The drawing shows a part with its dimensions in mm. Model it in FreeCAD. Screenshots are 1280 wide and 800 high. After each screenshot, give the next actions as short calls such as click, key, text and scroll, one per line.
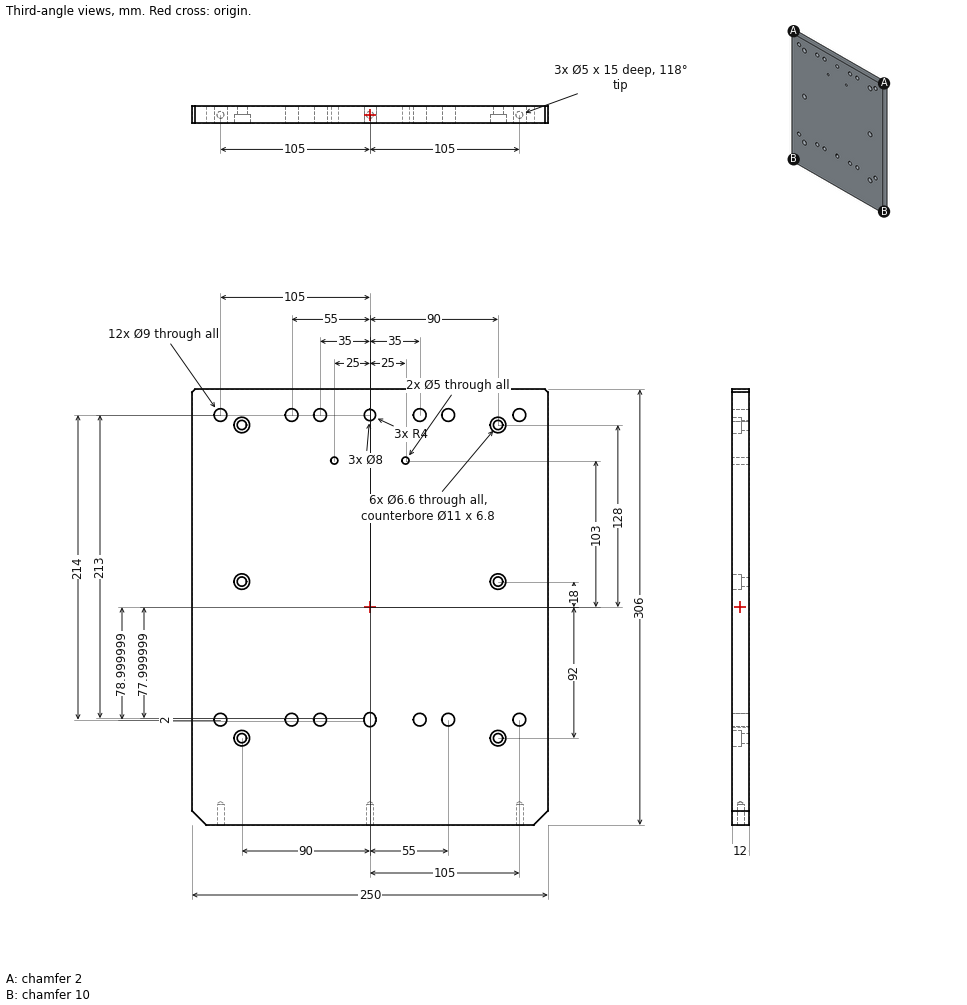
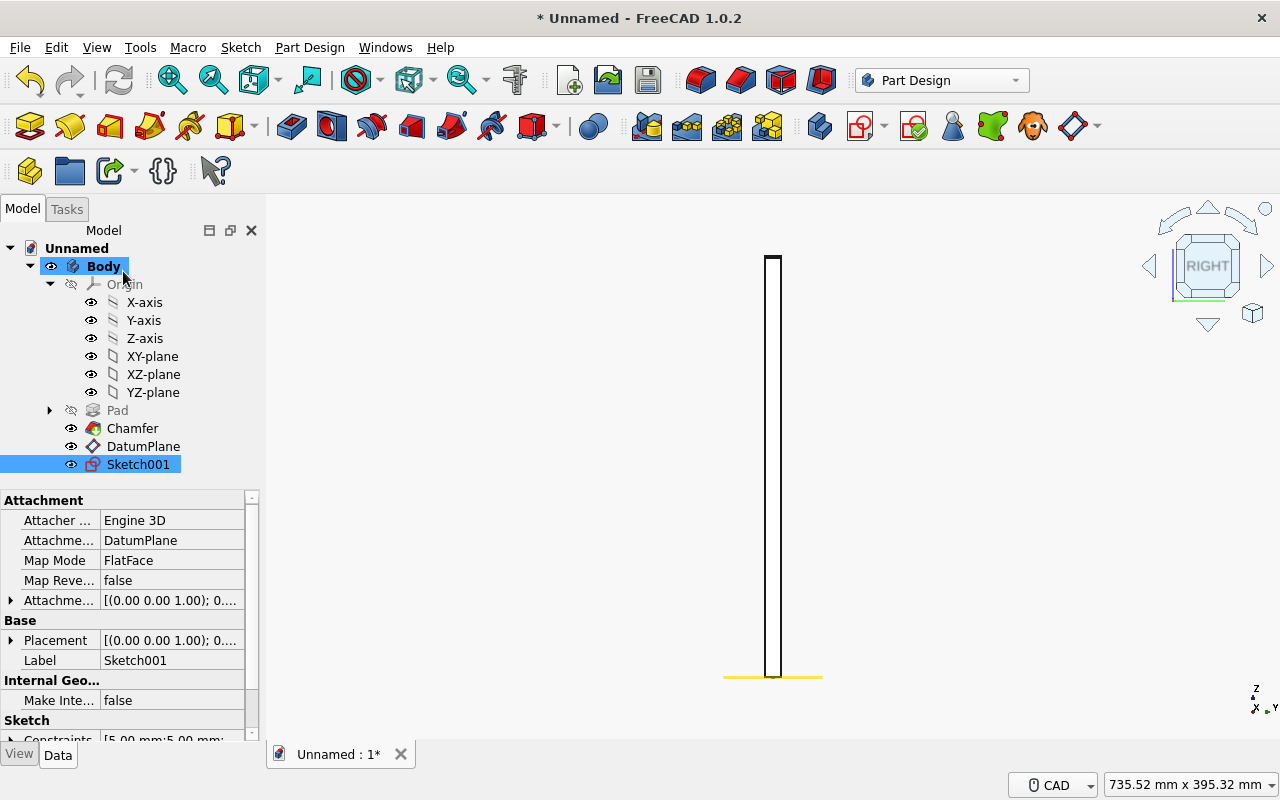
click(332, 126)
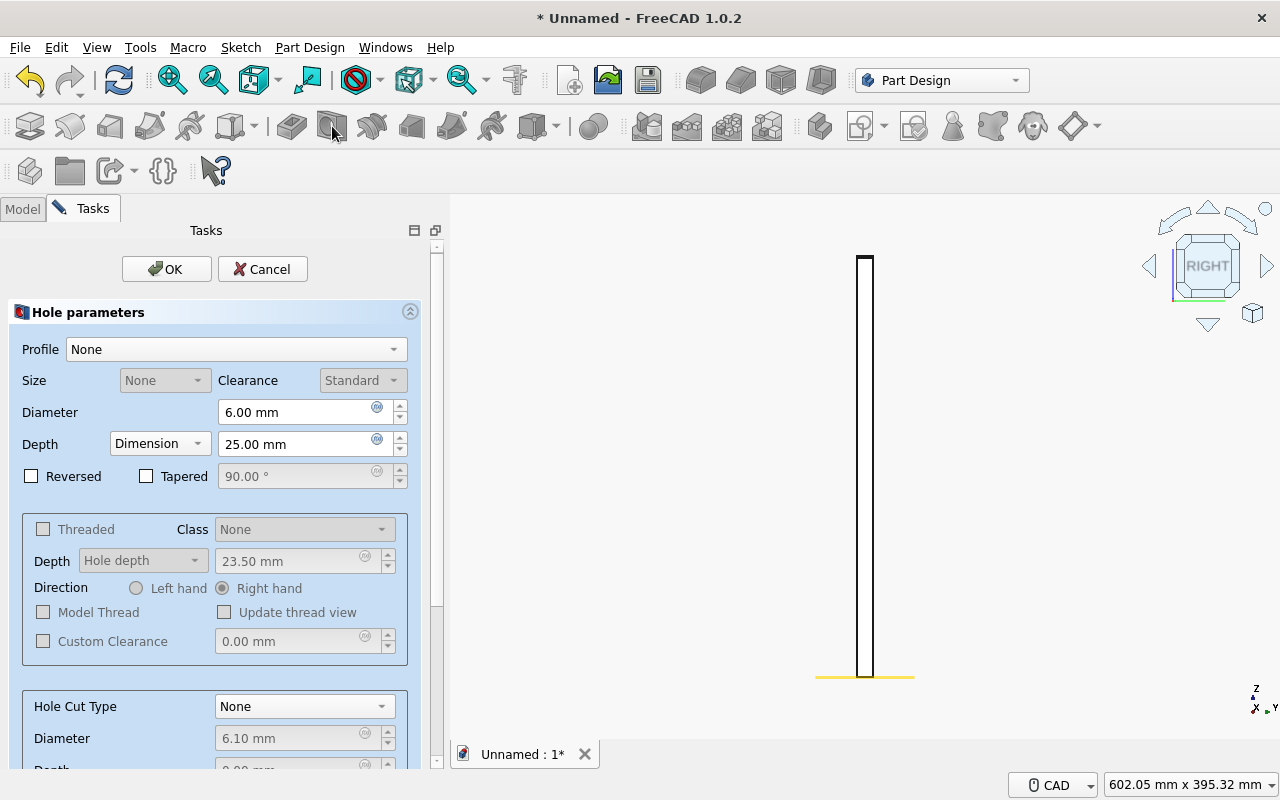
triple_click(305, 412)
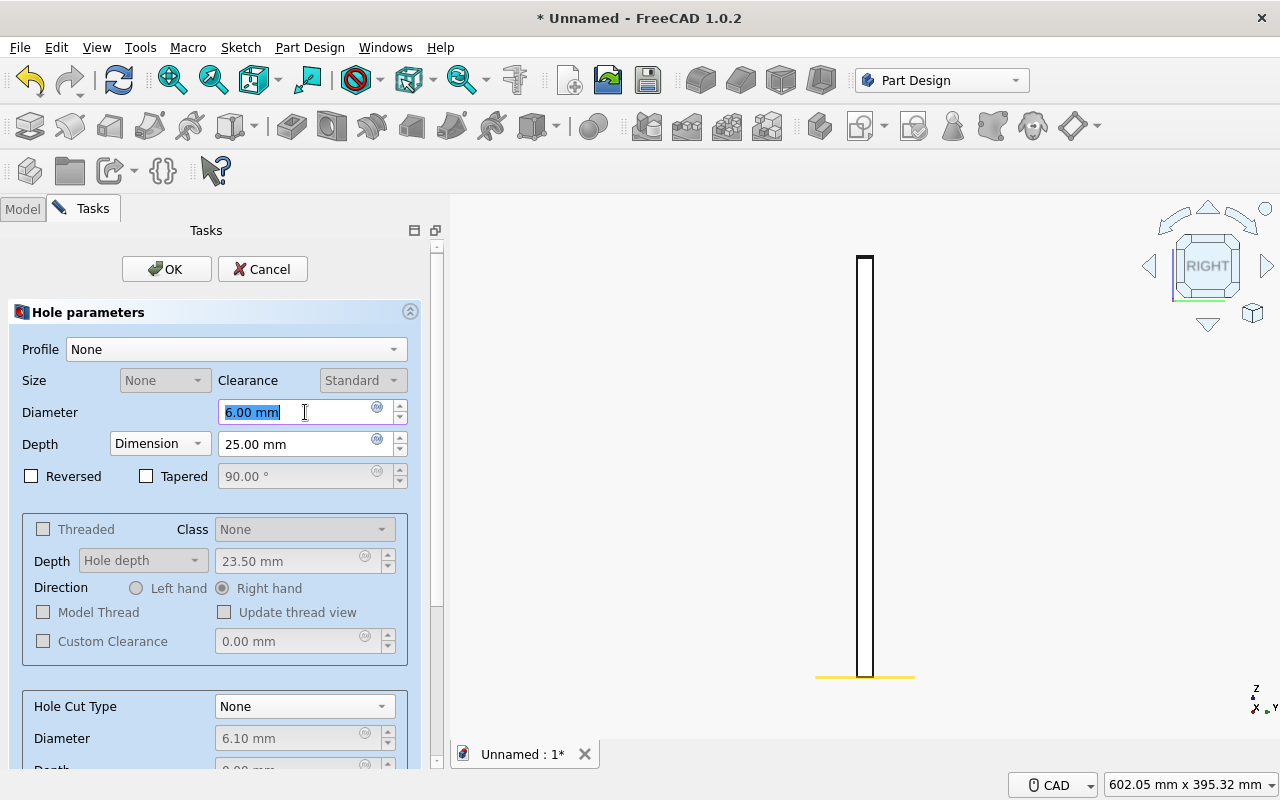
text(5)
key(Tab)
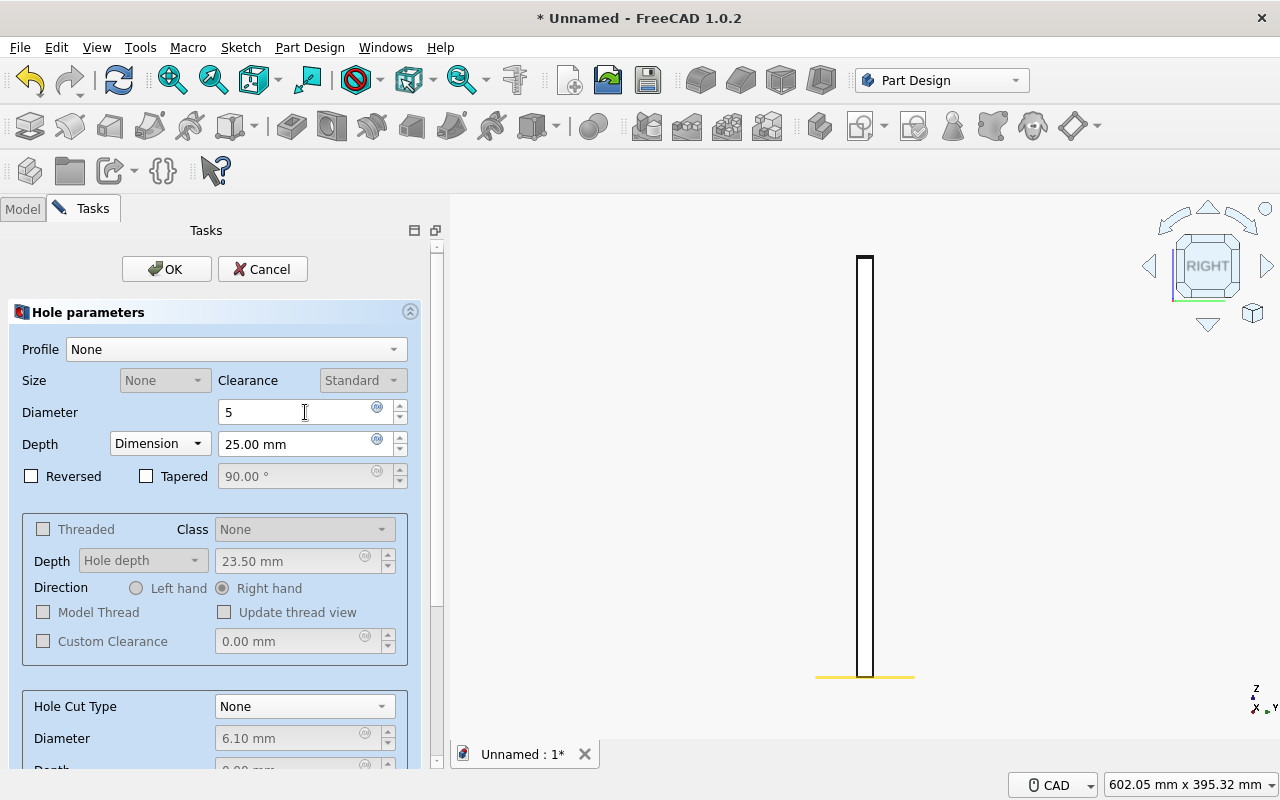
triple_click(305, 444)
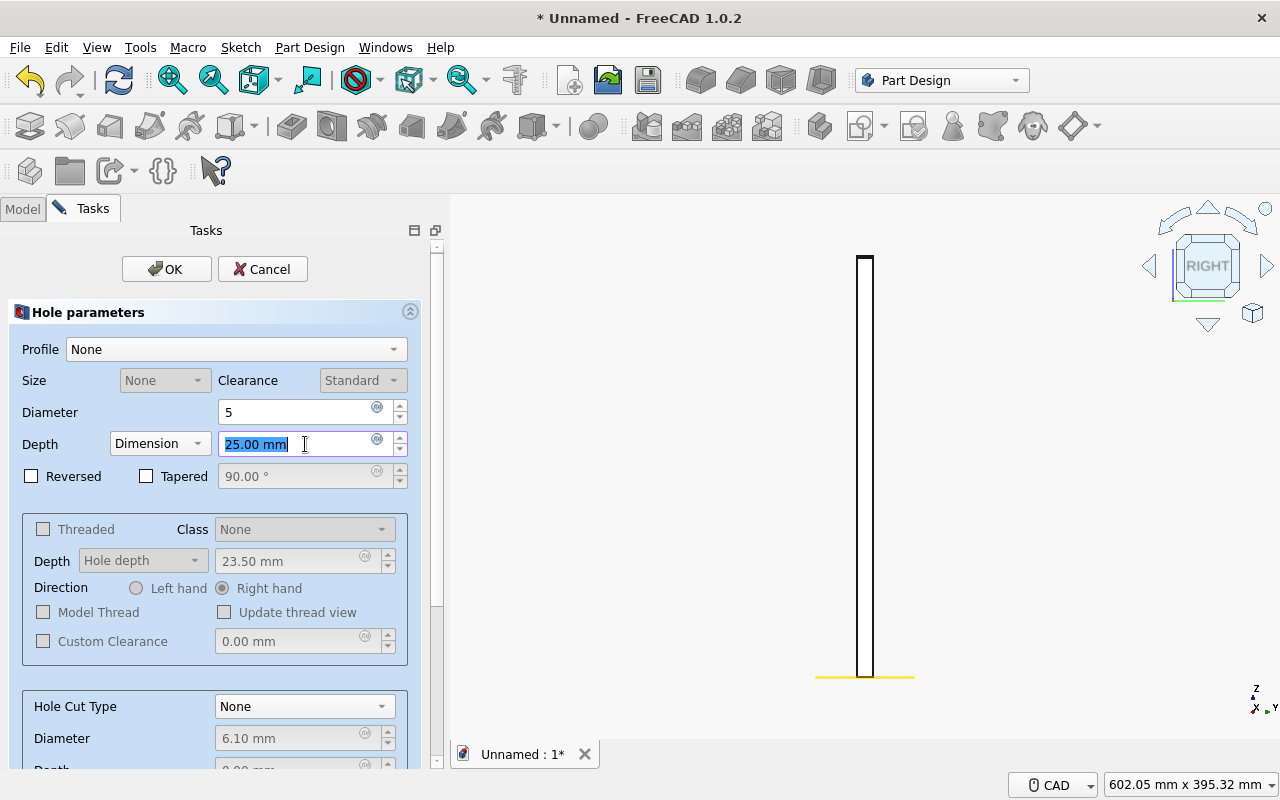
text(15)
key(Tab)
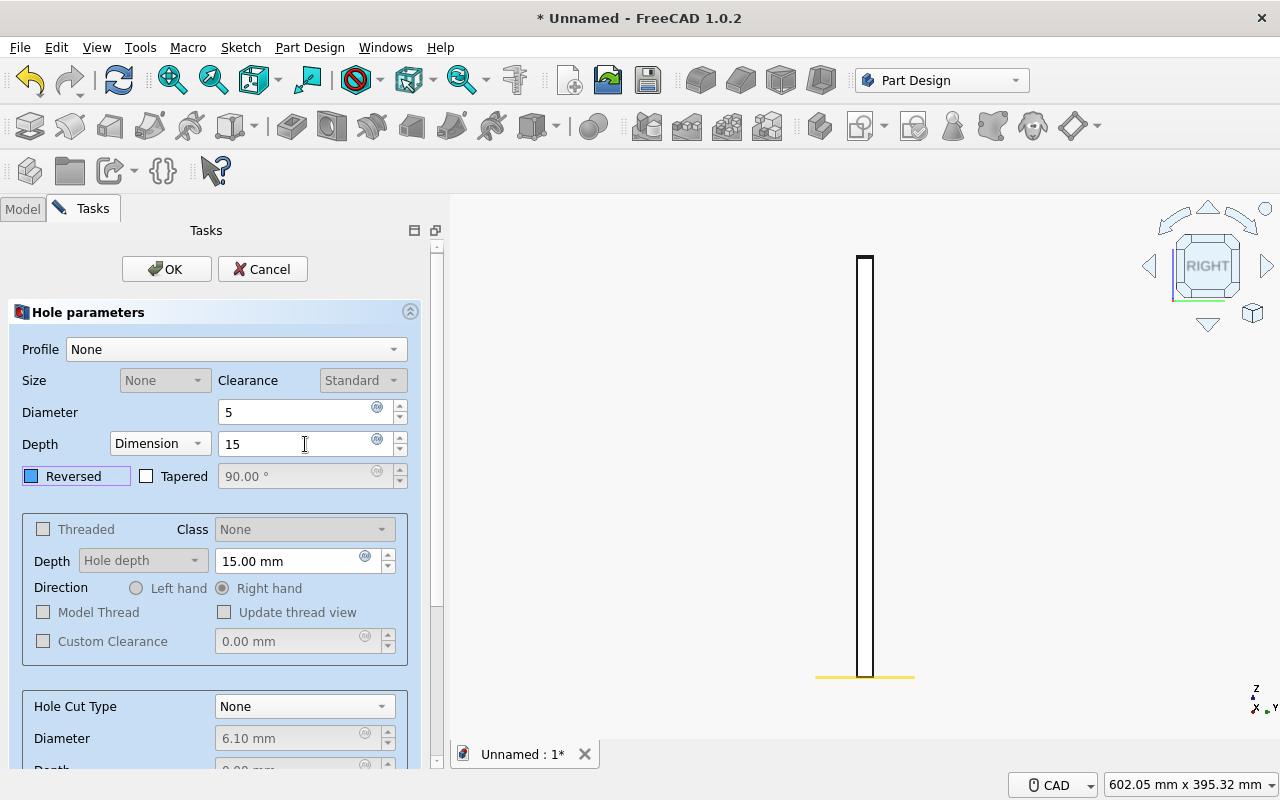
click(30, 476)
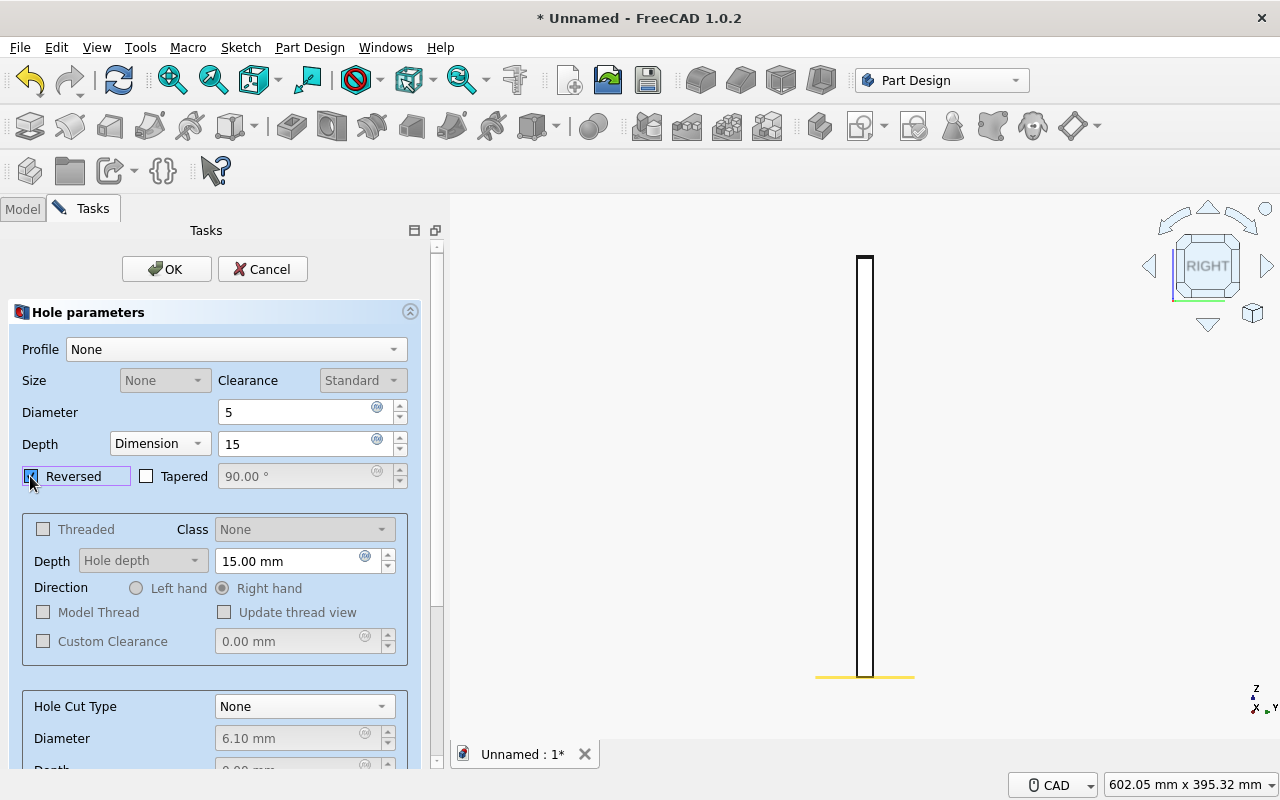
click(167, 269)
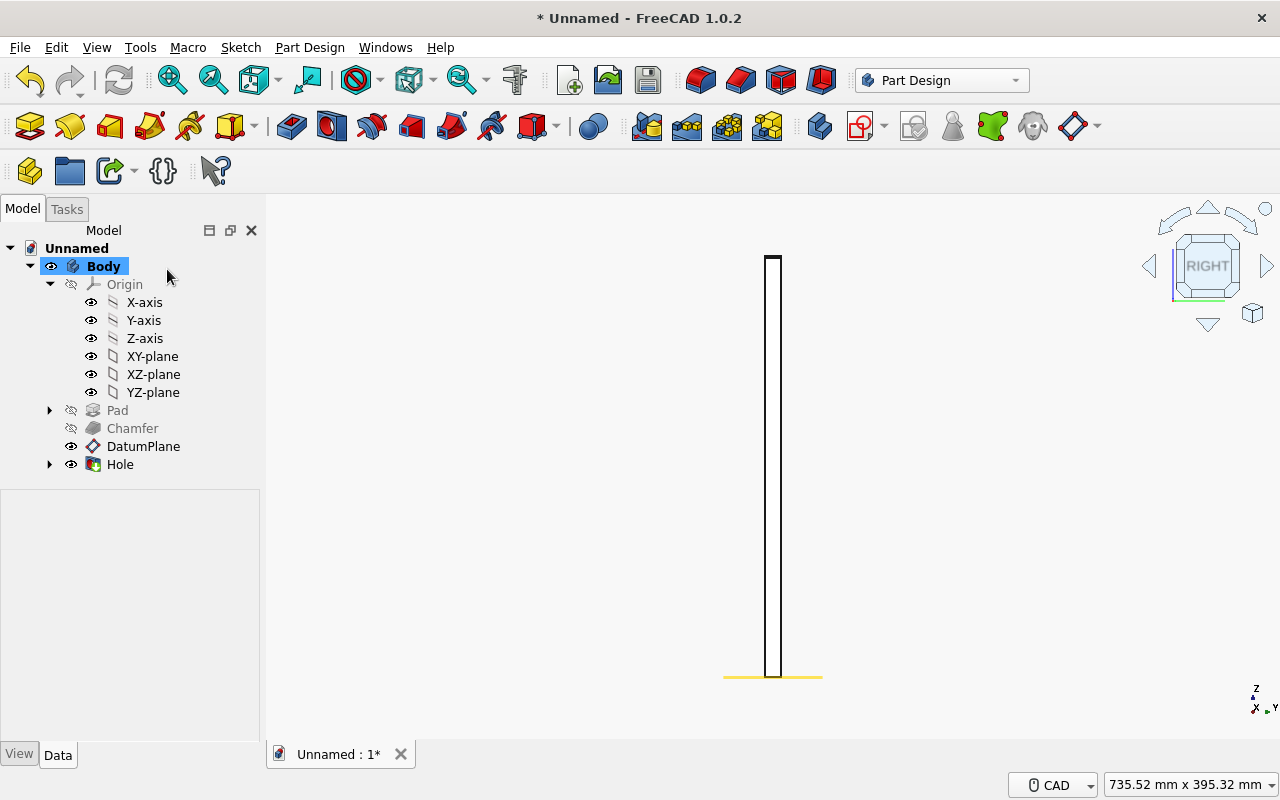
click(116, 446)
key(space)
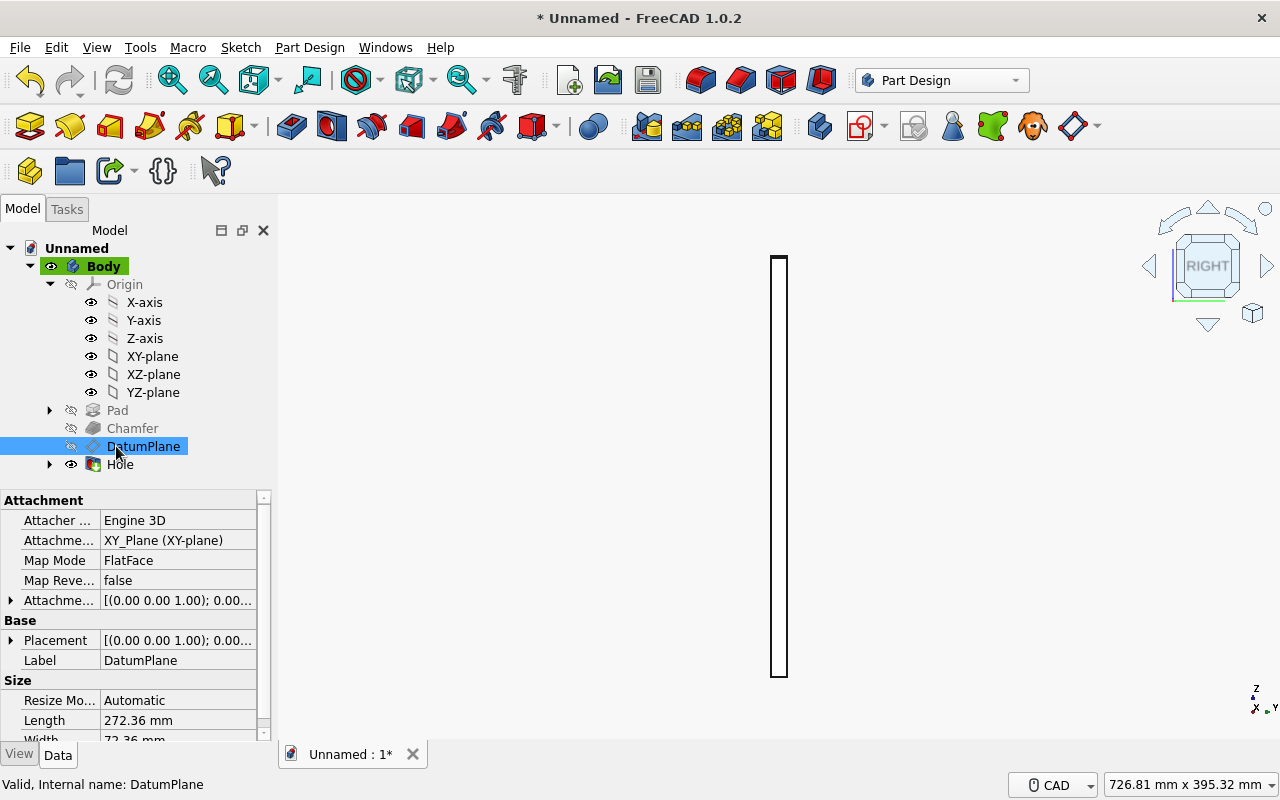
key(4)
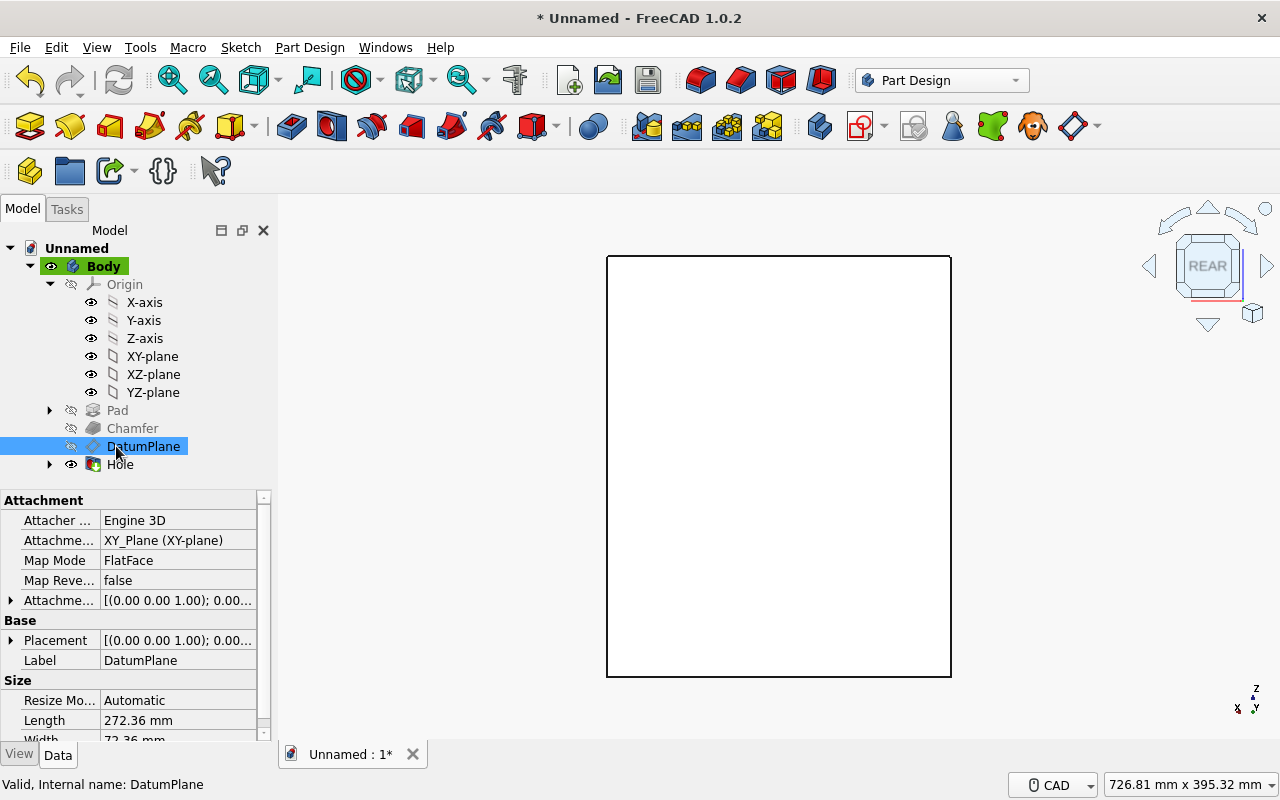
click(779, 466)